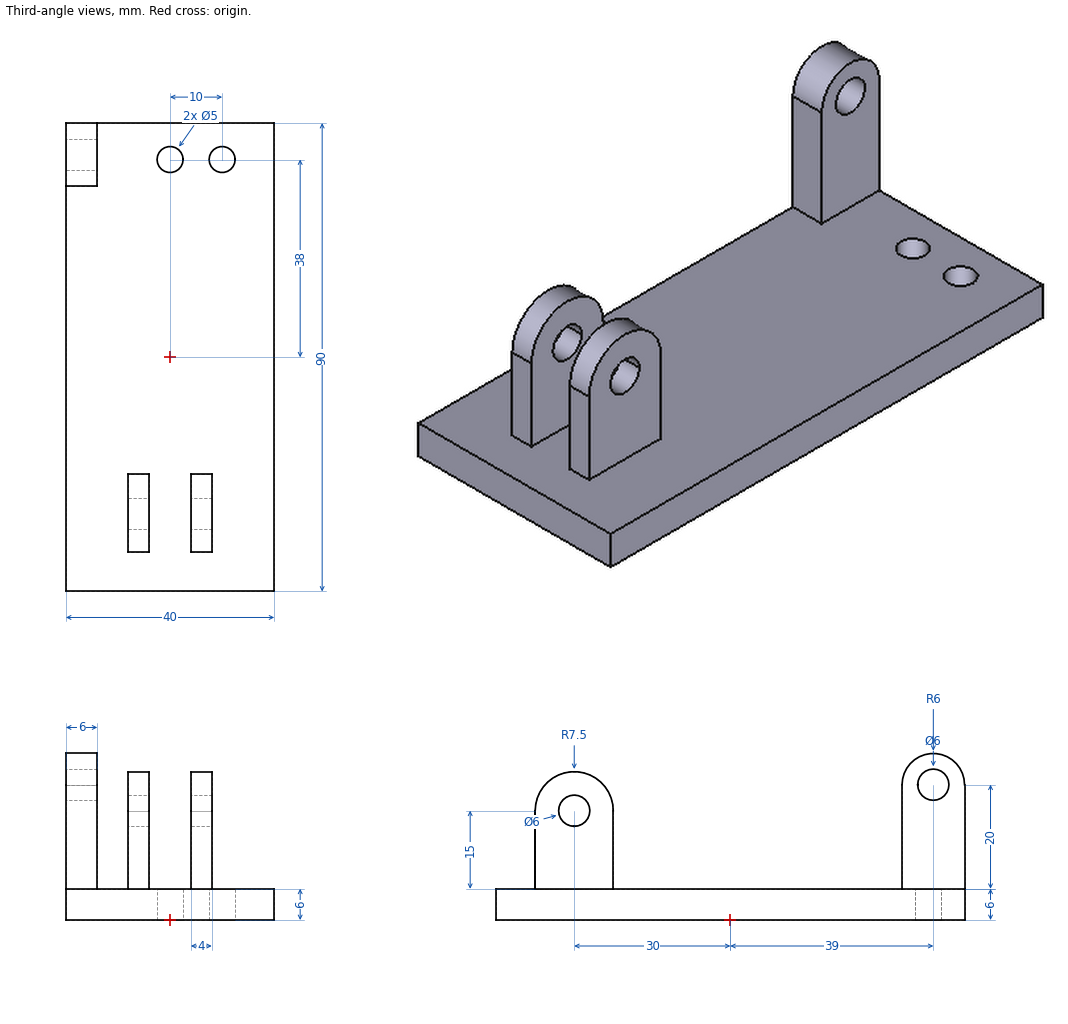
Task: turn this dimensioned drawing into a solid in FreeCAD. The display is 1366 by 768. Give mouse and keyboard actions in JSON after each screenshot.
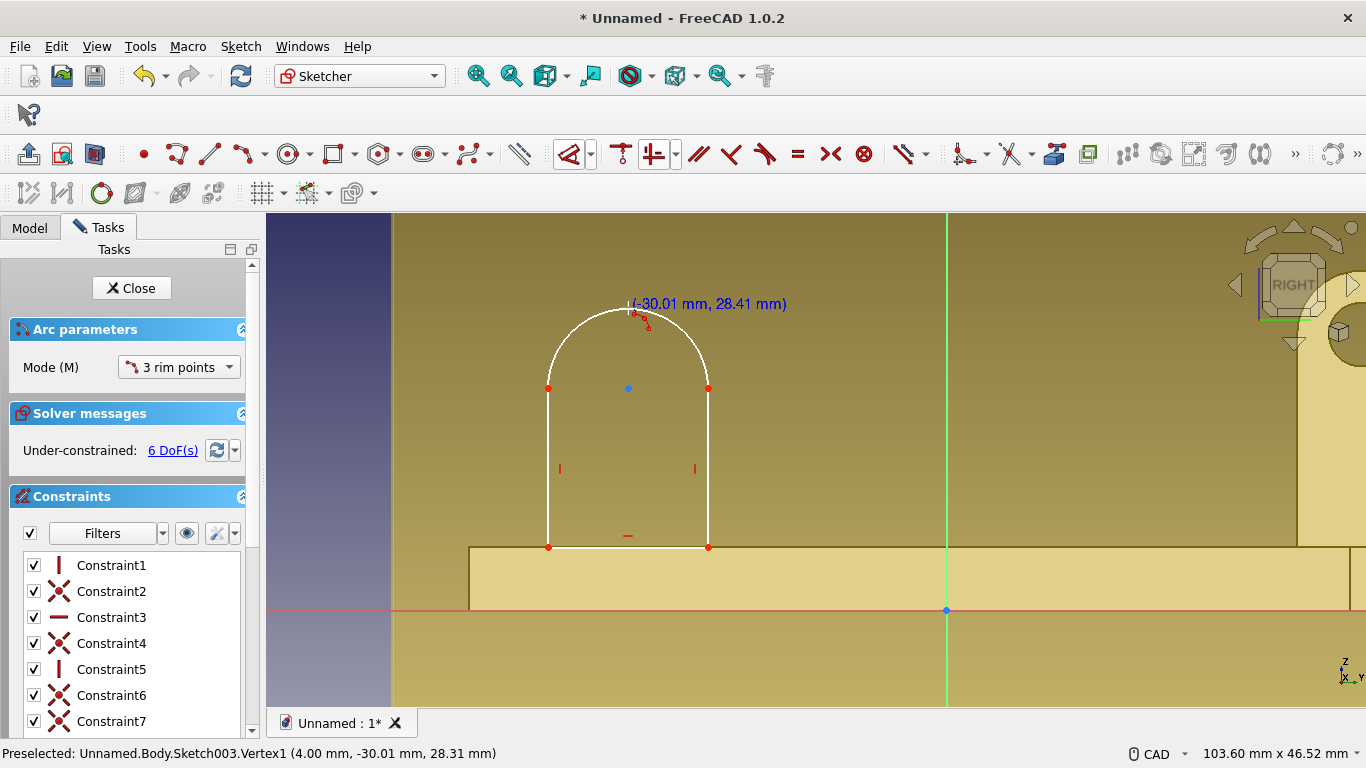
{"action": "left_click", "coordinate": [288, 154]}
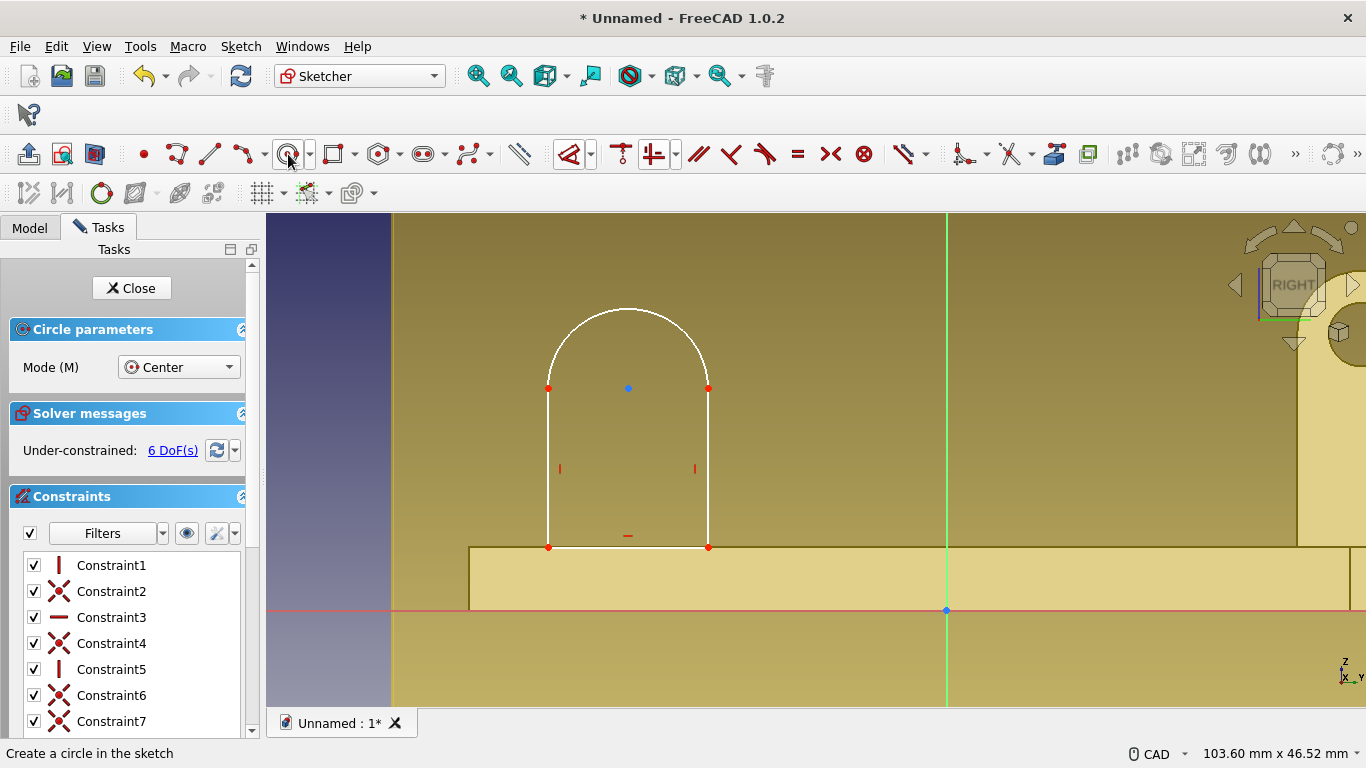
{"action": "left_click", "coordinate": [628, 388]}
{"action": "mouse_move", "coordinate": [651, 365]}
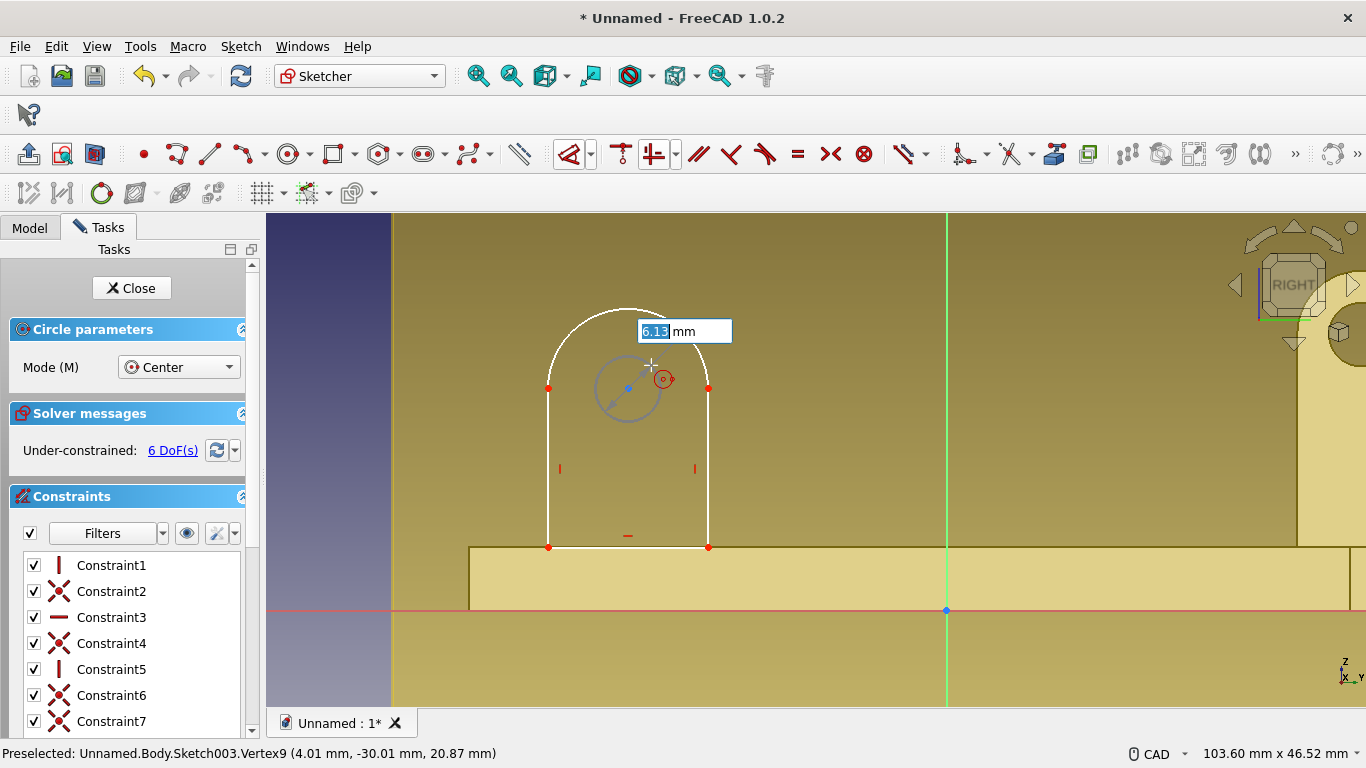
{"action": "type", "text": "6"}
{"action": "key", "text": "Return"}
{"action": "key", "text": "Escape"}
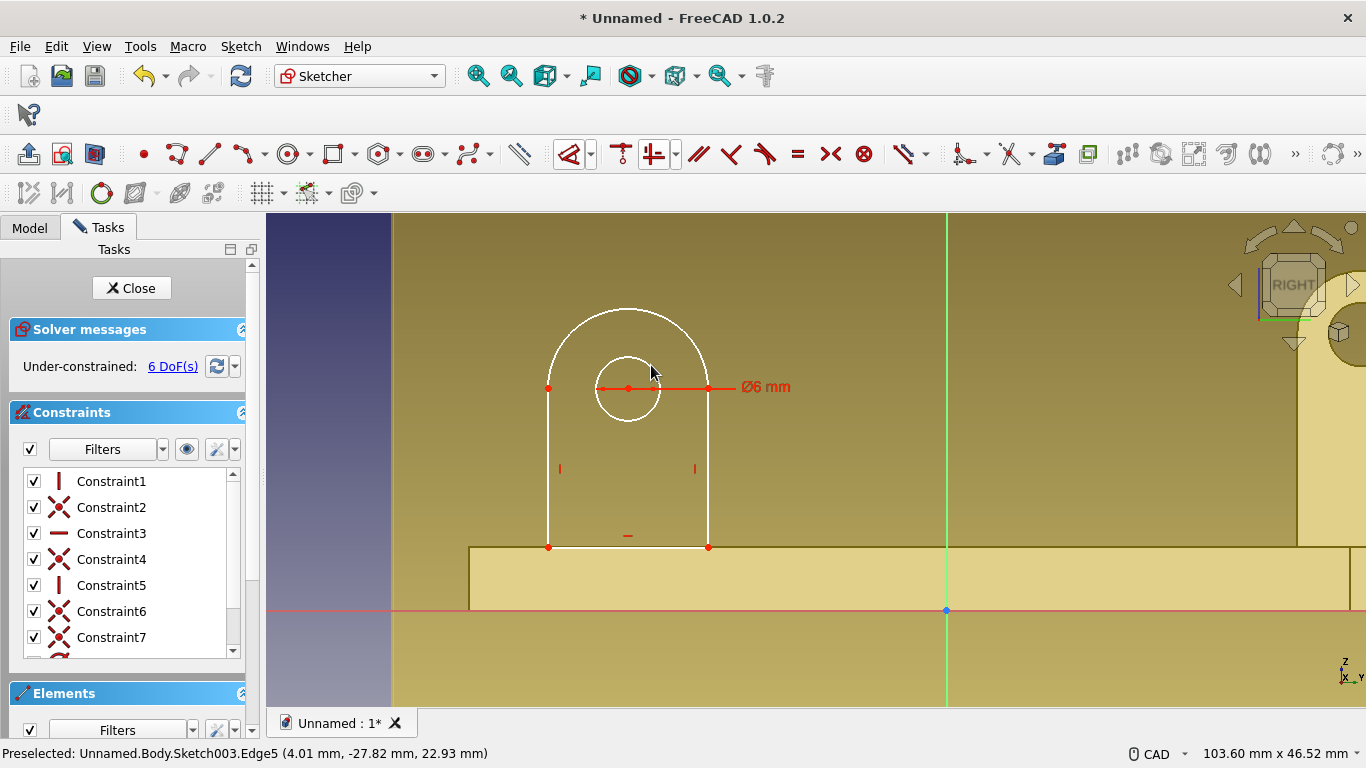
{"action": "left_click", "coordinate": [548, 437]}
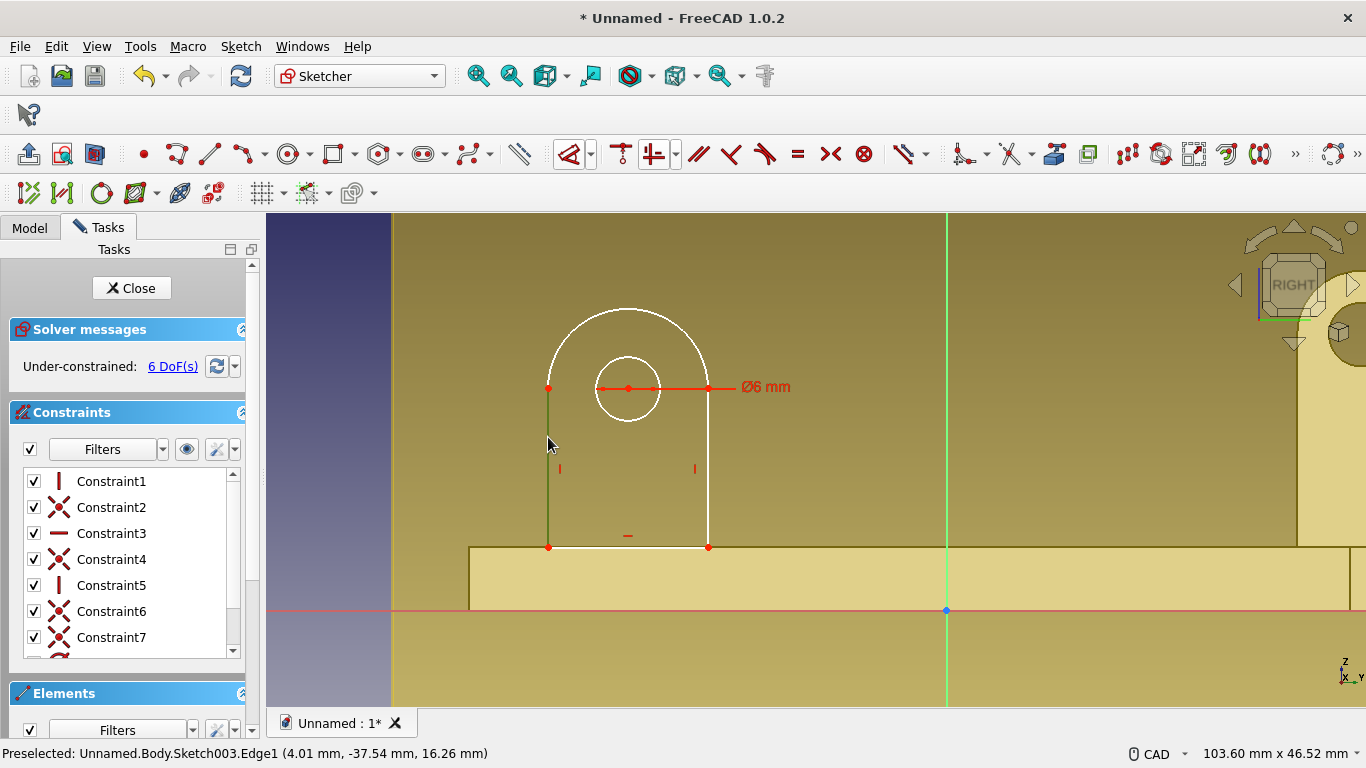
{"action": "left_click", "coordinate": [675, 324]}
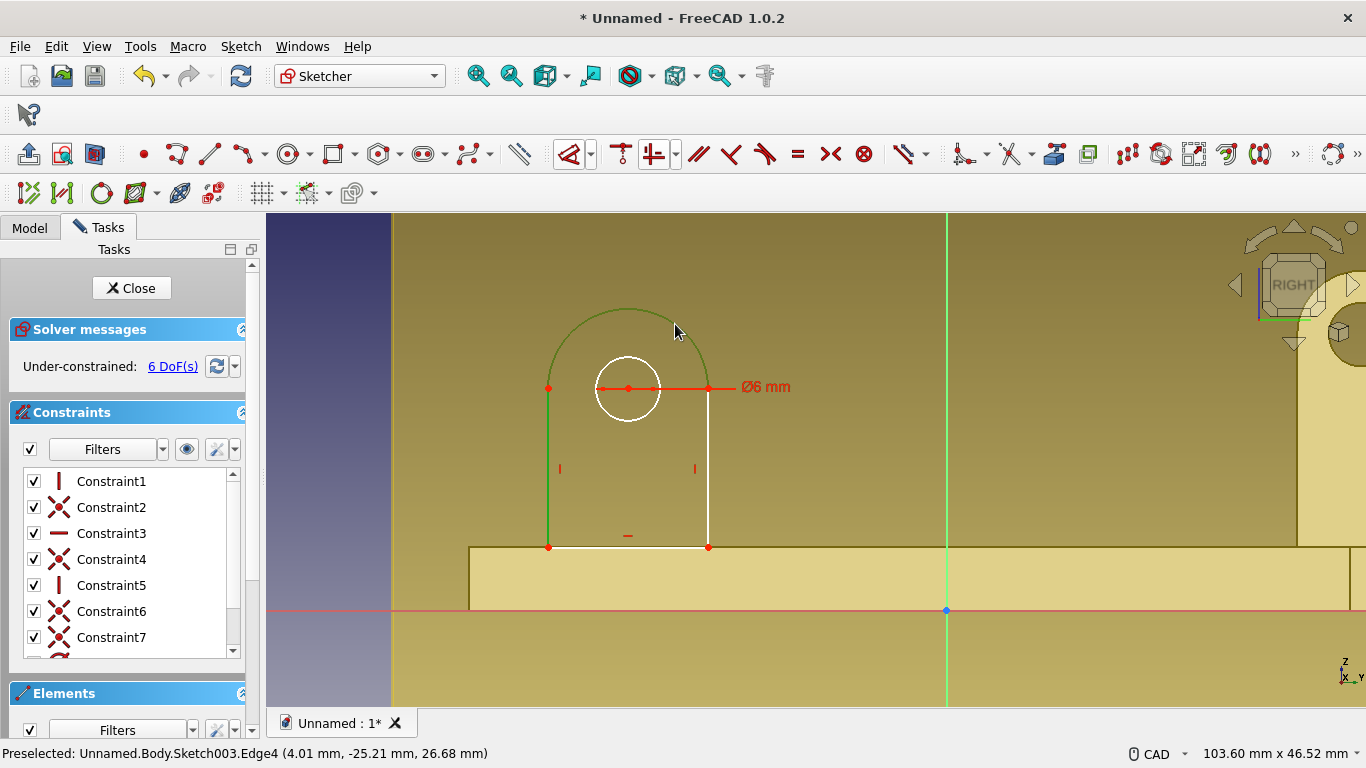
{"action": "left_click", "coordinate": [765, 154]}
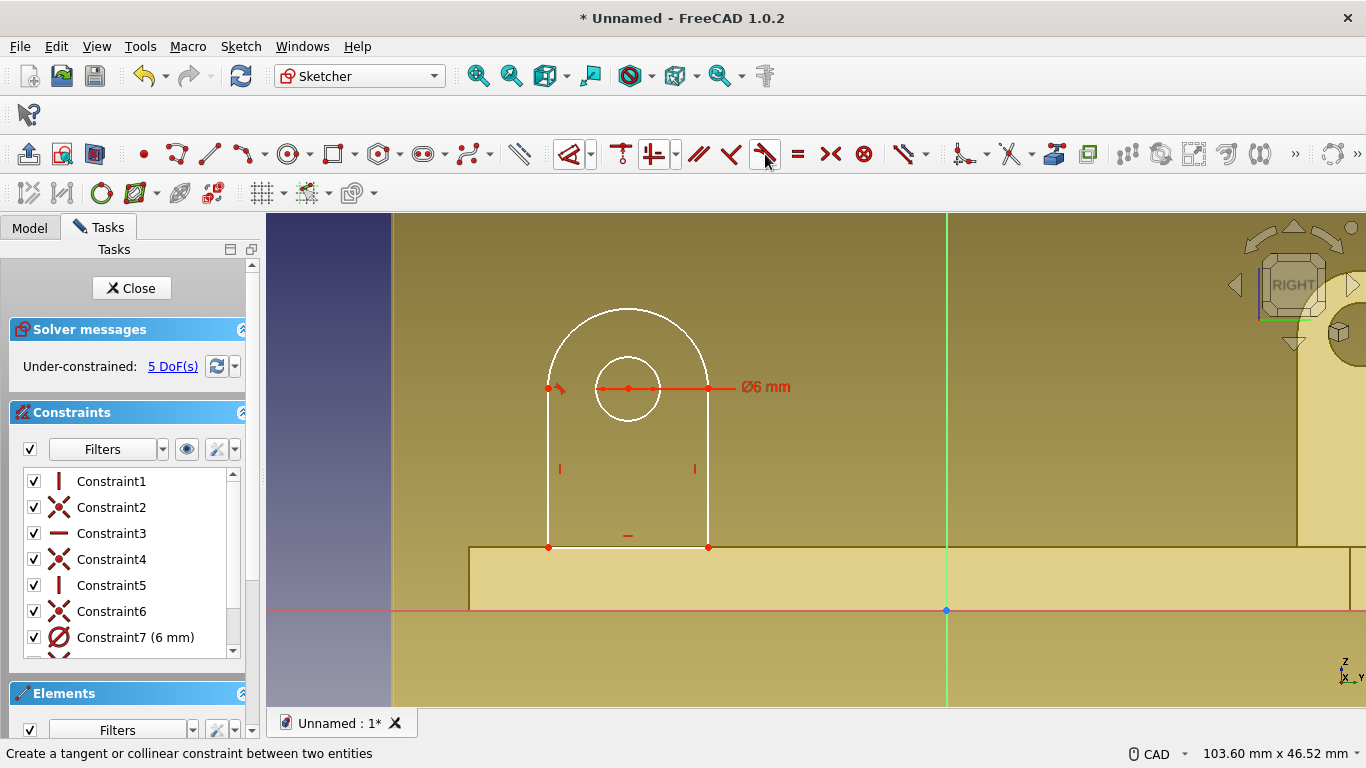
{"action": "left_click", "coordinate": [708, 500]}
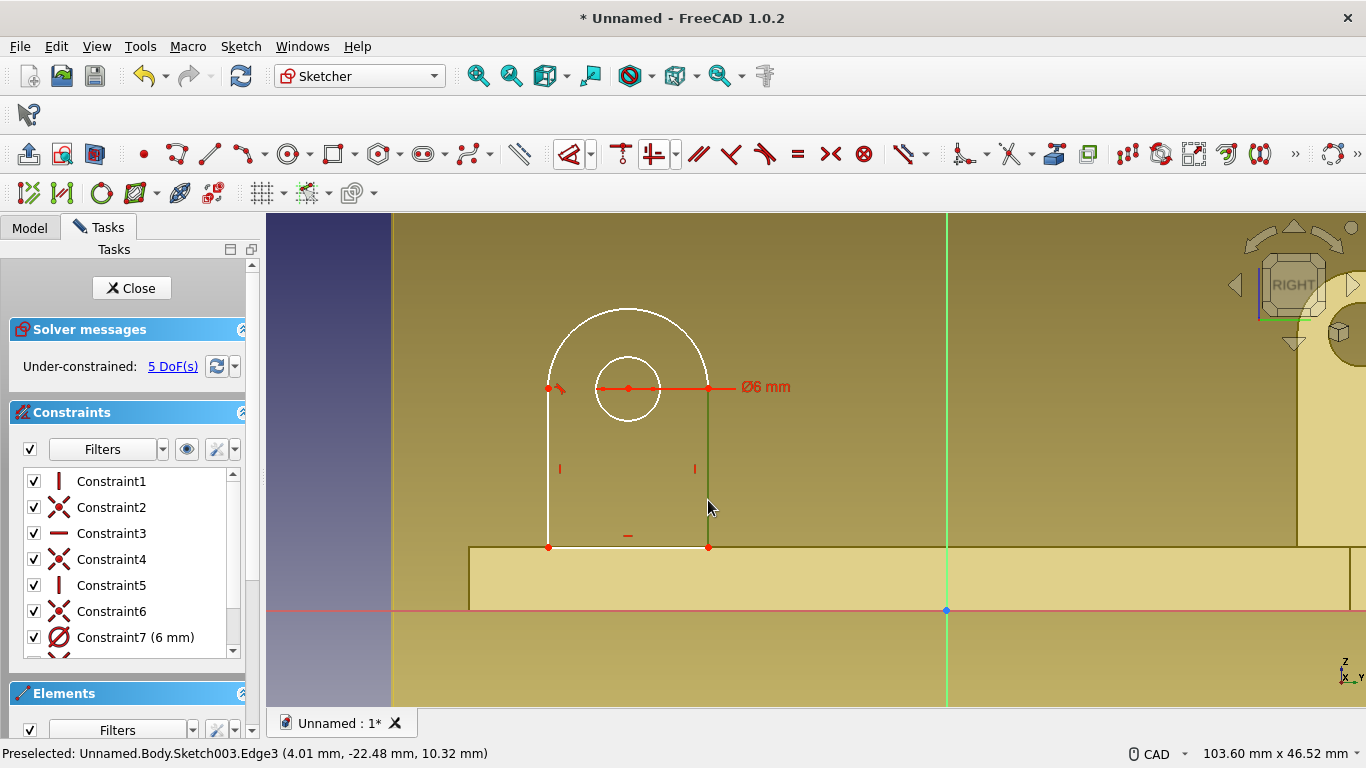
{"action": "left_click", "coordinate": [675, 324]}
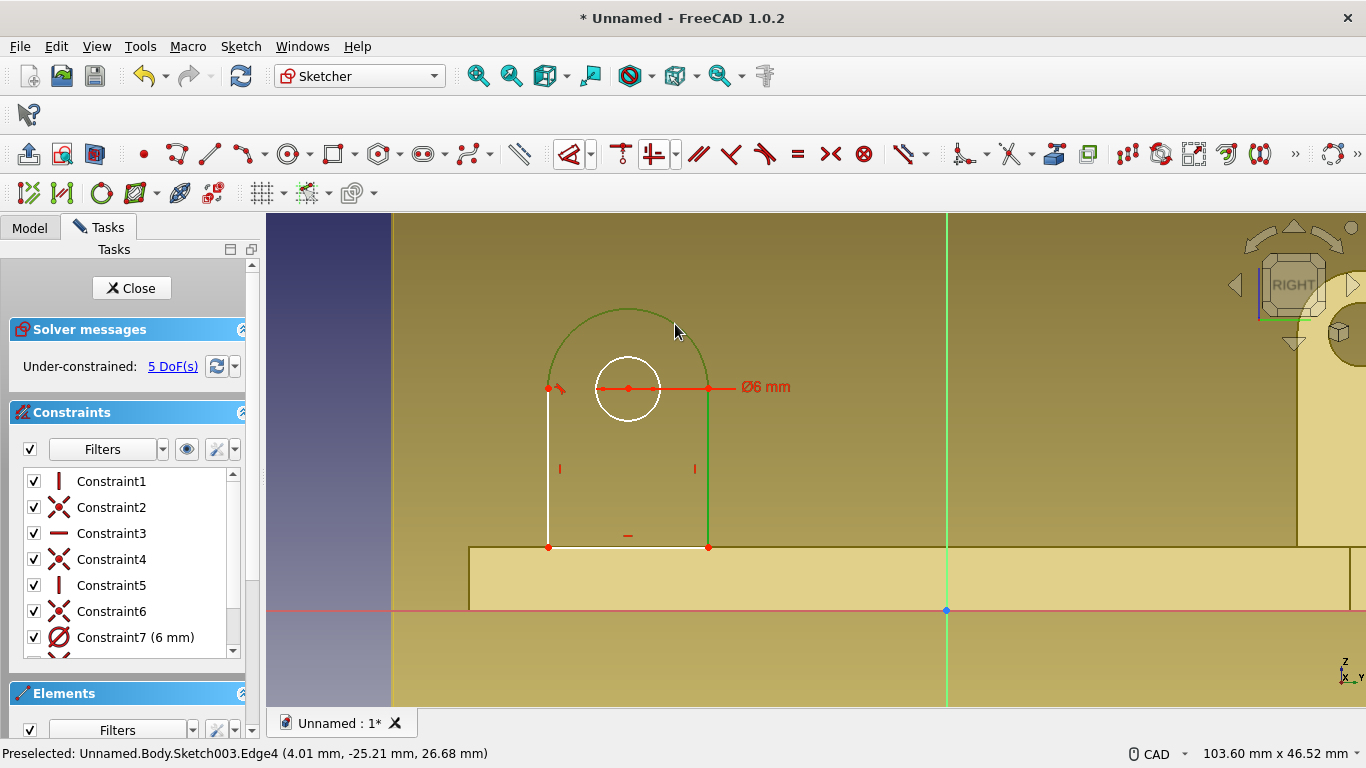
{"action": "left_click", "coordinate": [765, 154]}